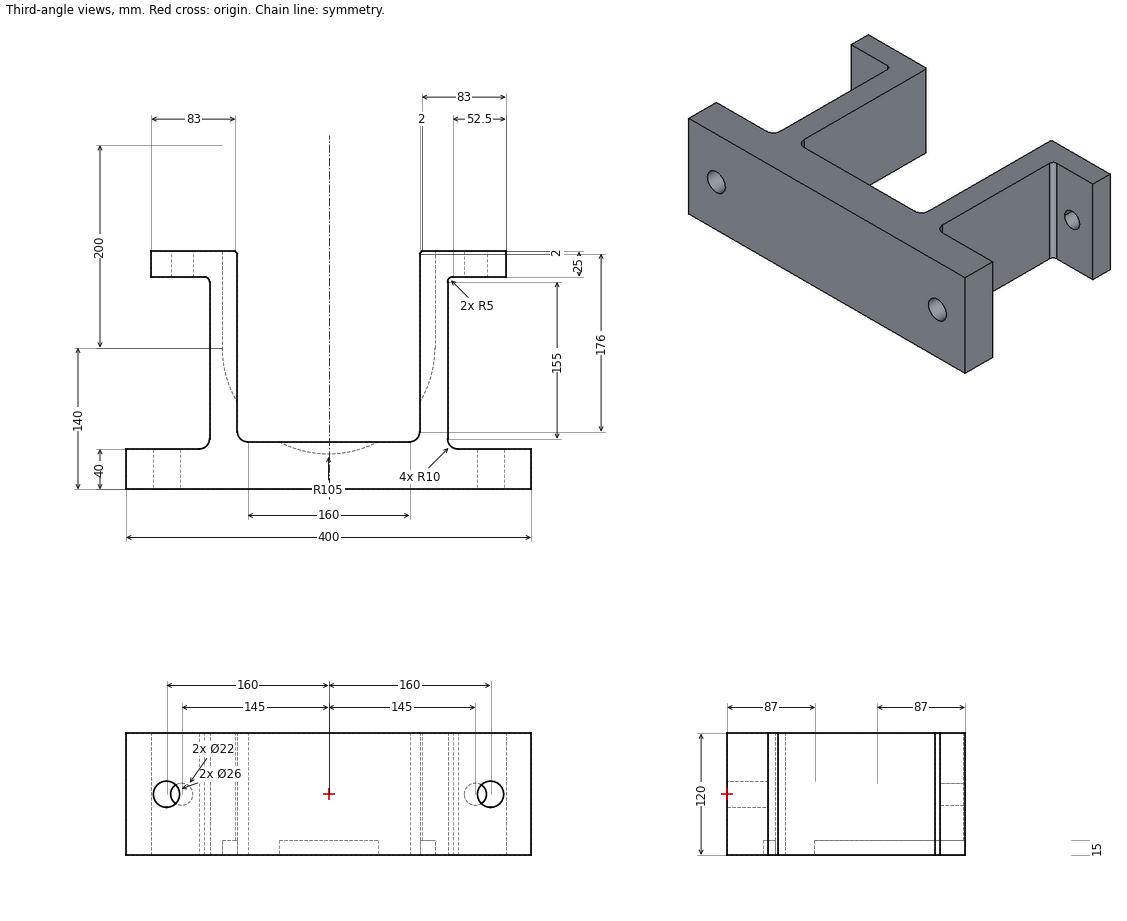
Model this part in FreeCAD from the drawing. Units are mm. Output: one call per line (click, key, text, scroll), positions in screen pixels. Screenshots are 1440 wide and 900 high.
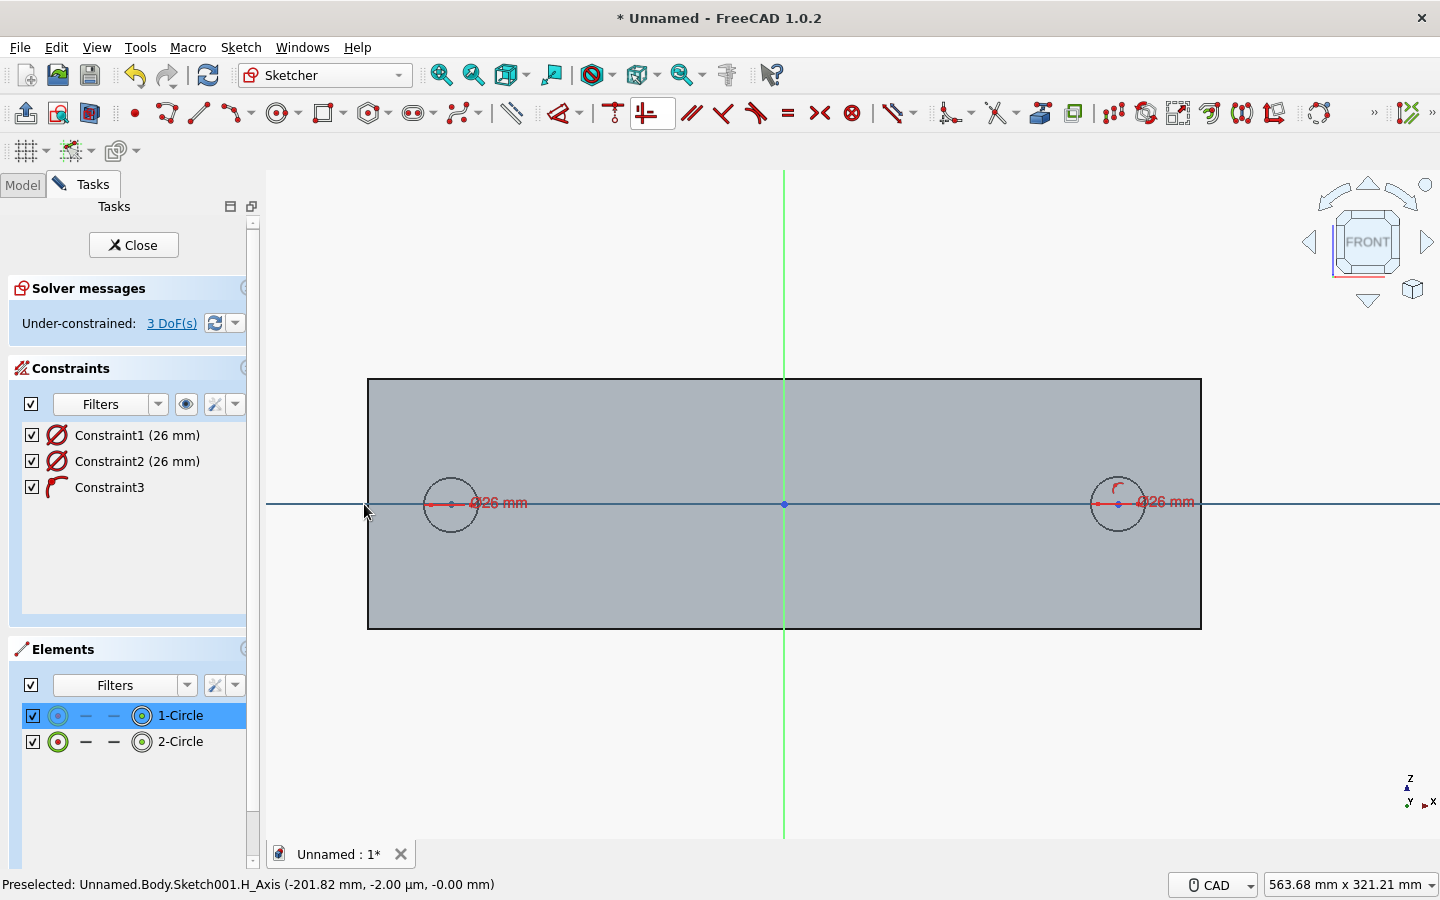
click(614, 114)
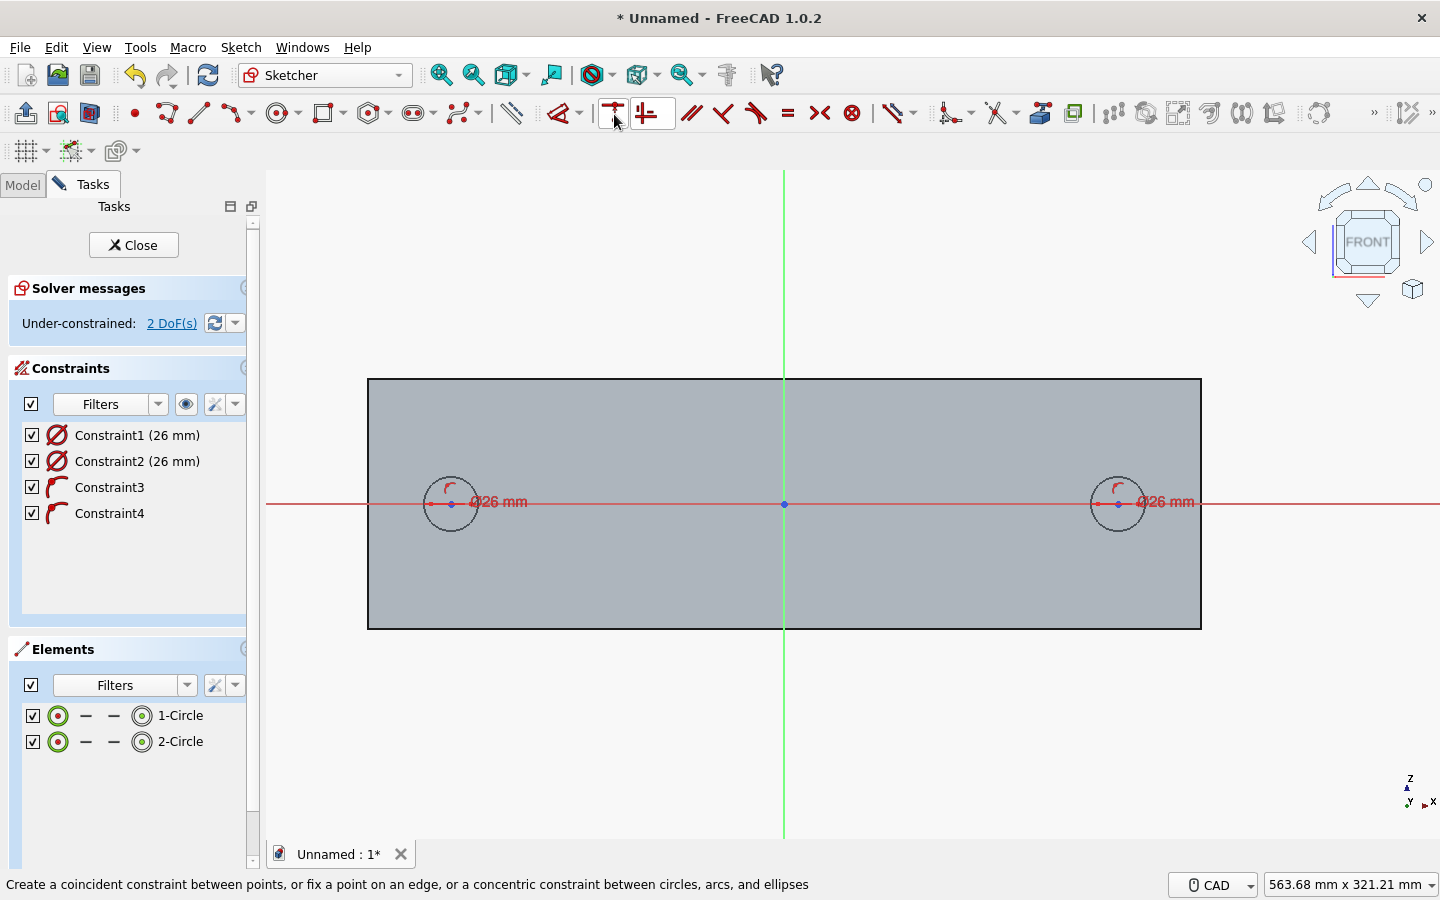
click(558, 114)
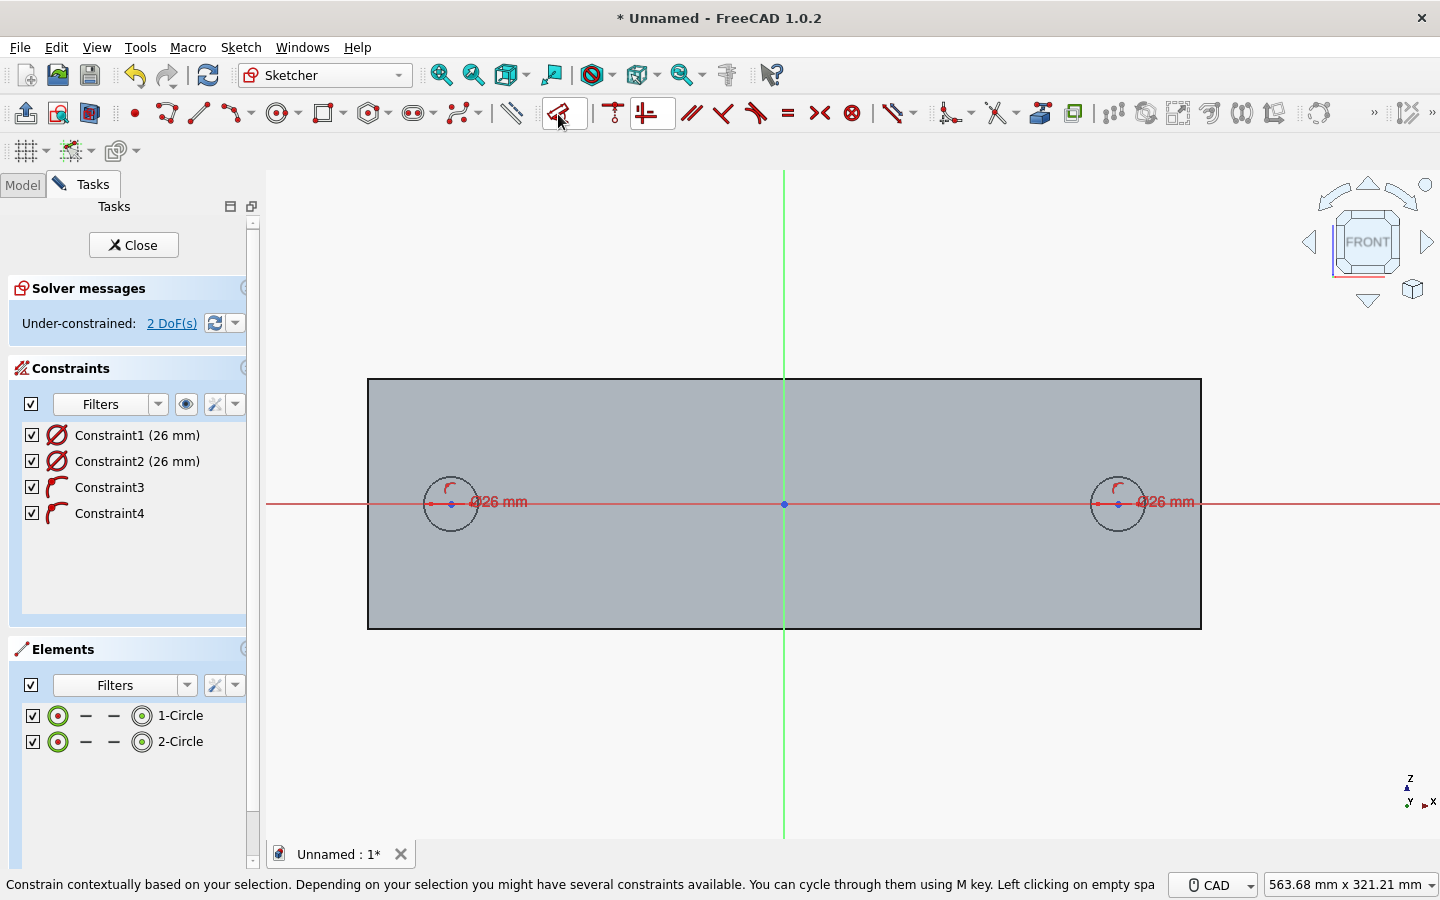
click(451, 504)
click(618, 538)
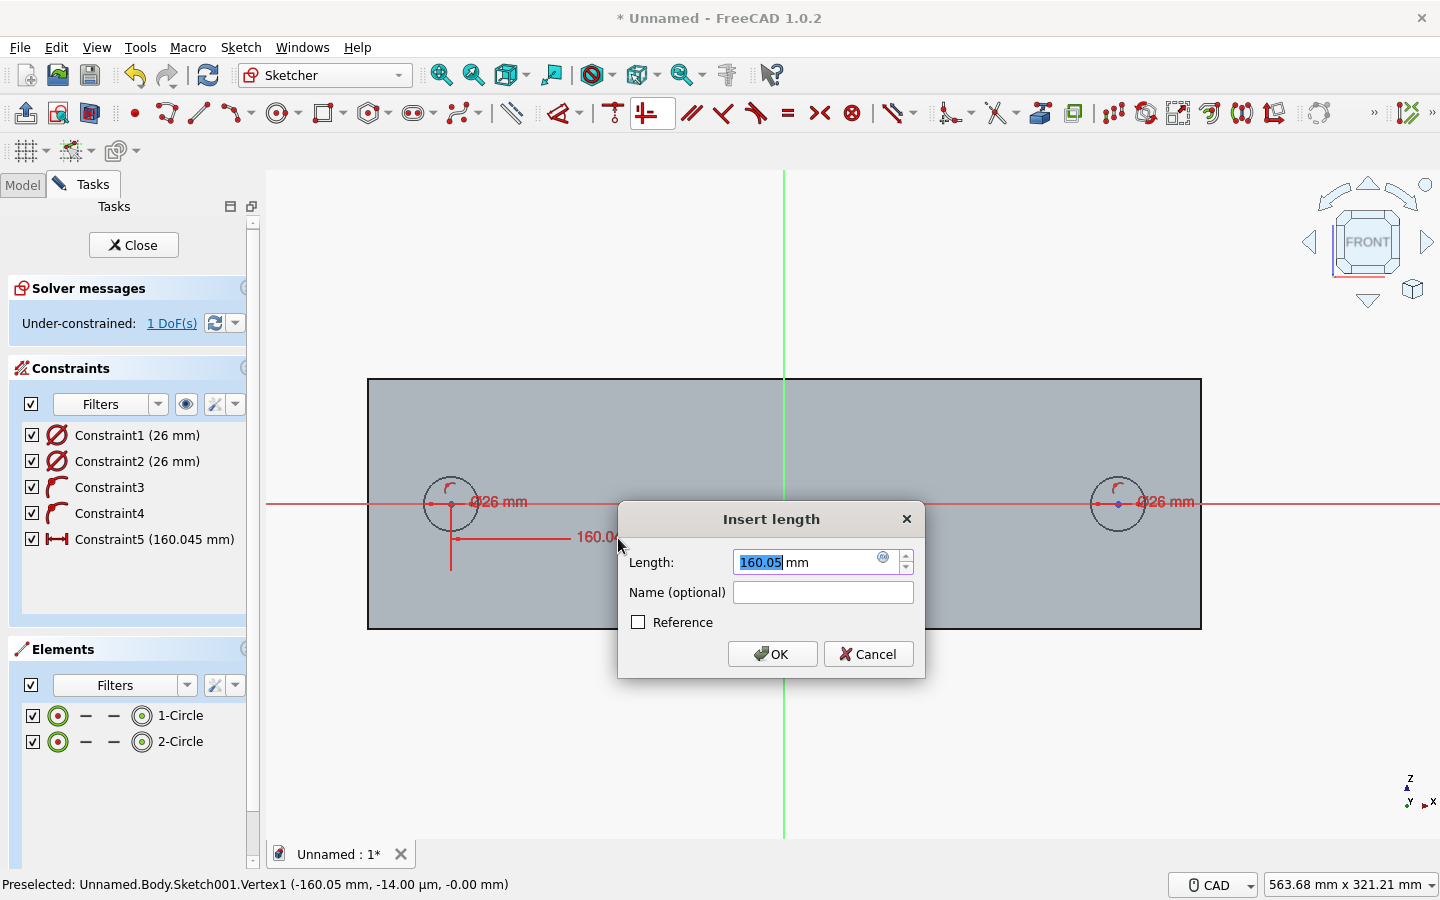
text(160)
key(Return)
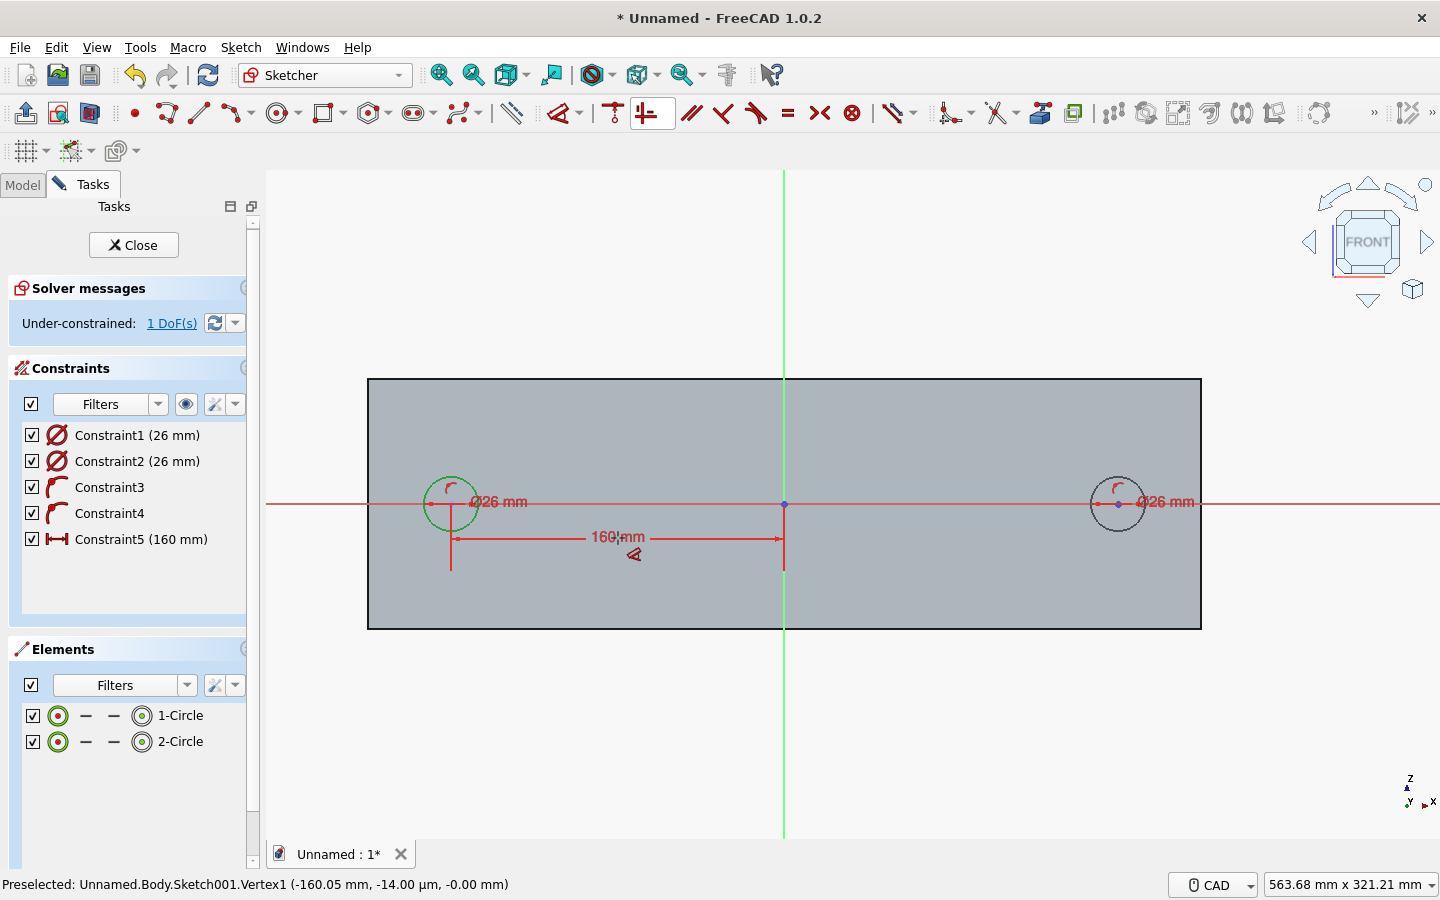
click(1118, 504)
click(951, 538)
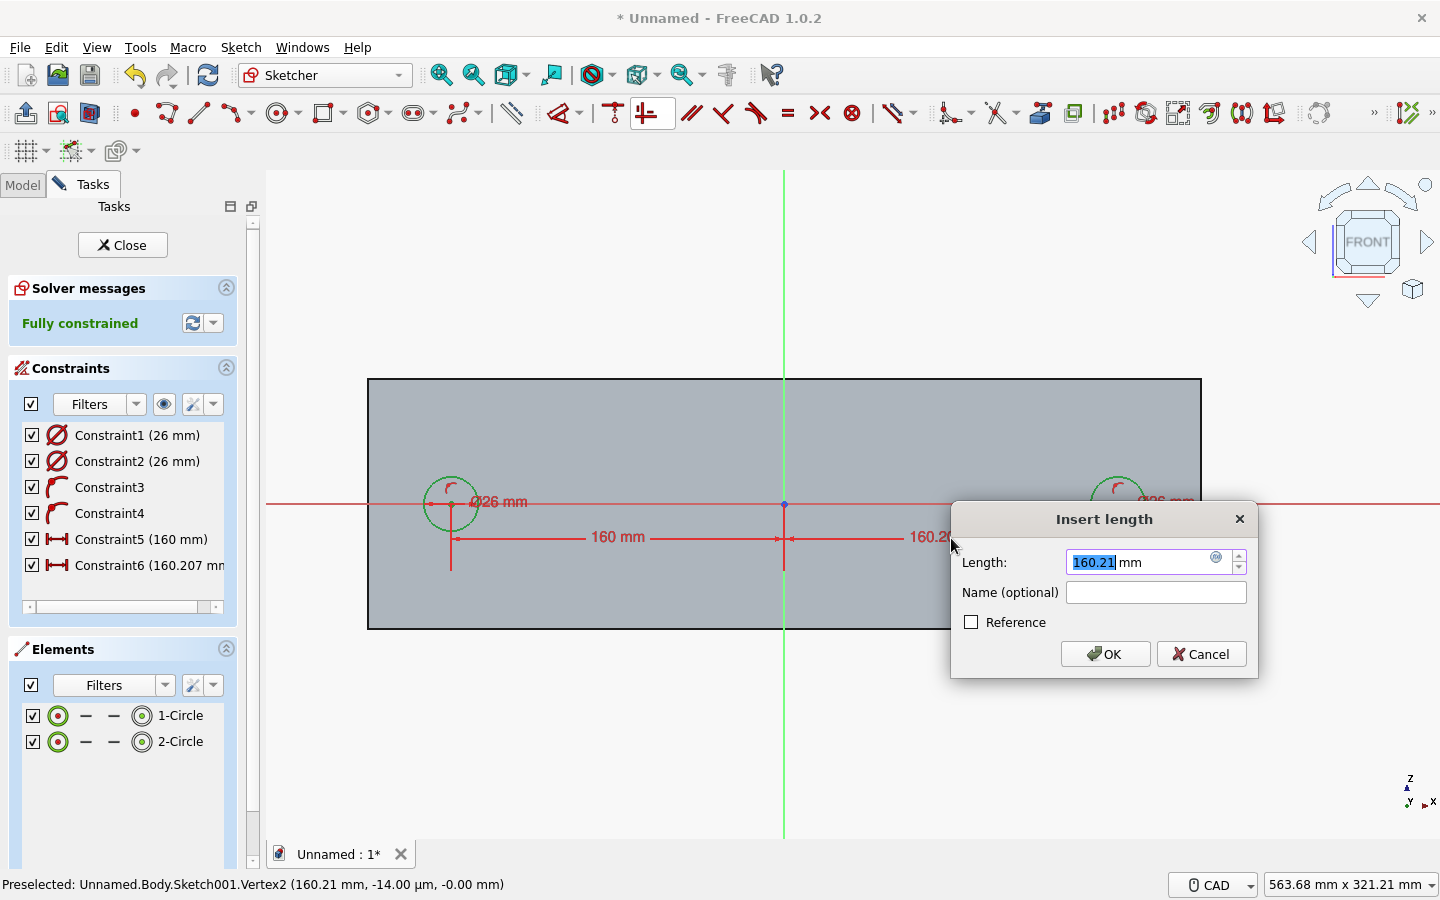
text(160)
key(Return)
key(Escape)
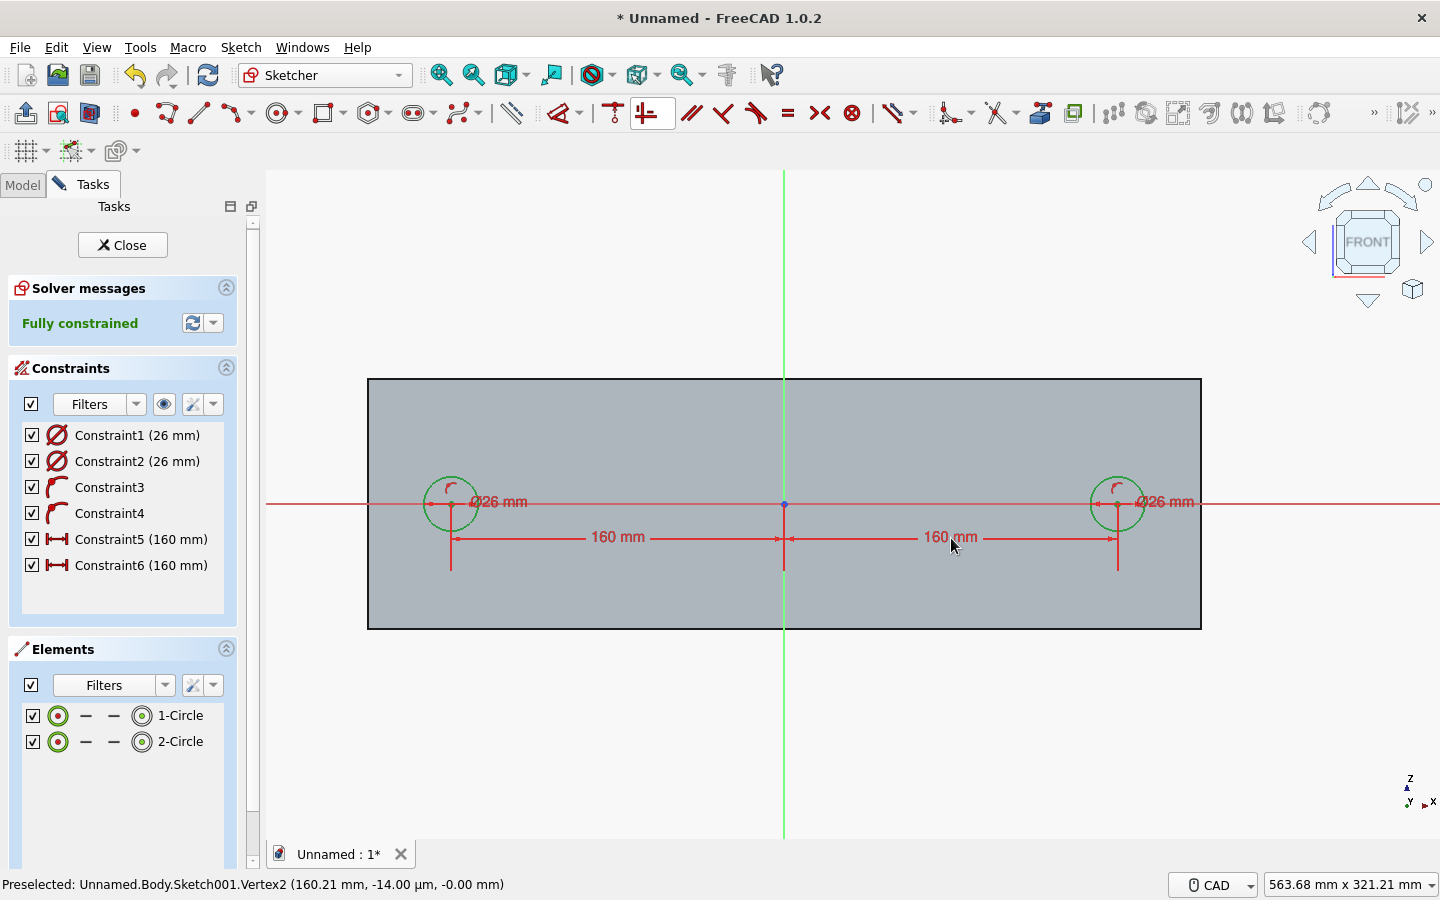
click(123, 245)